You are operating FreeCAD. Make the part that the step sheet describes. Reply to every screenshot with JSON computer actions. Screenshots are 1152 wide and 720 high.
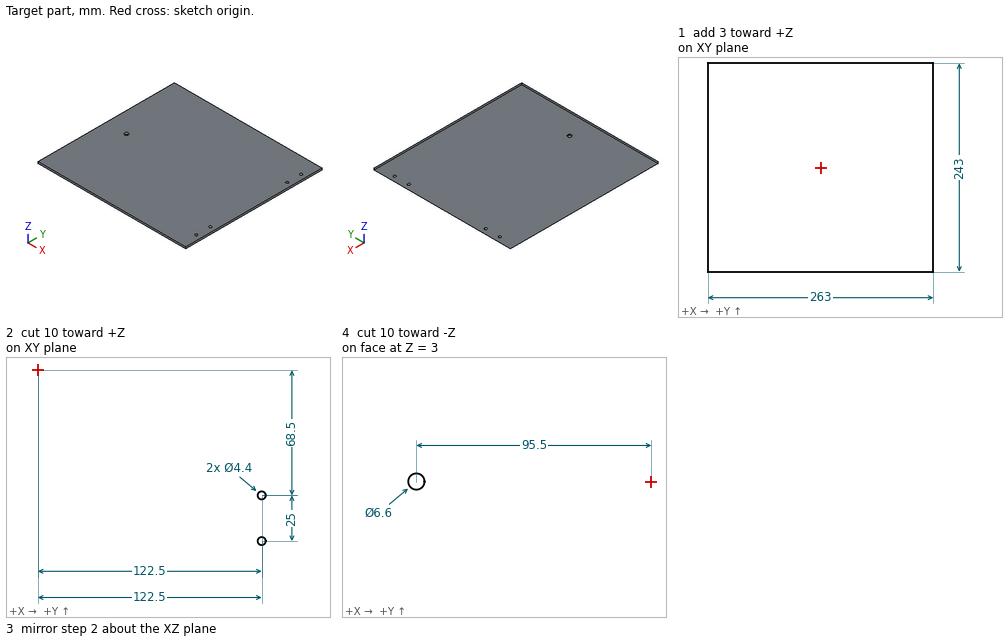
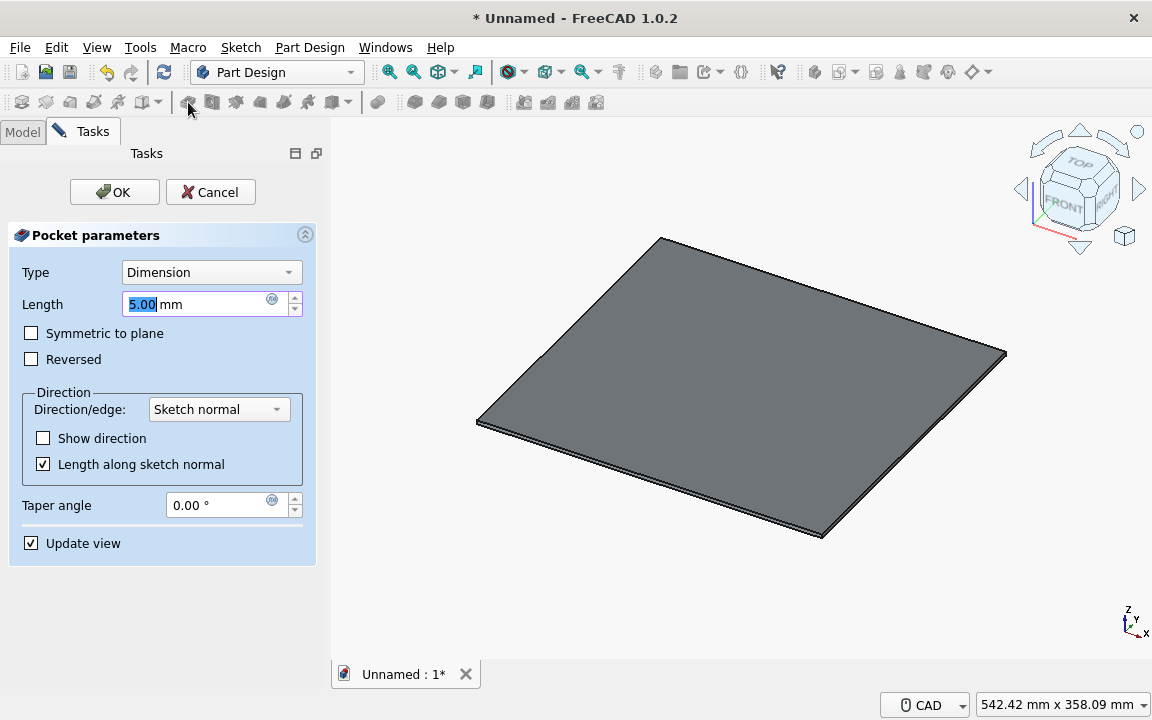
{"action": "type", "text": "10"}
{"action": "key", "text": "Tab"}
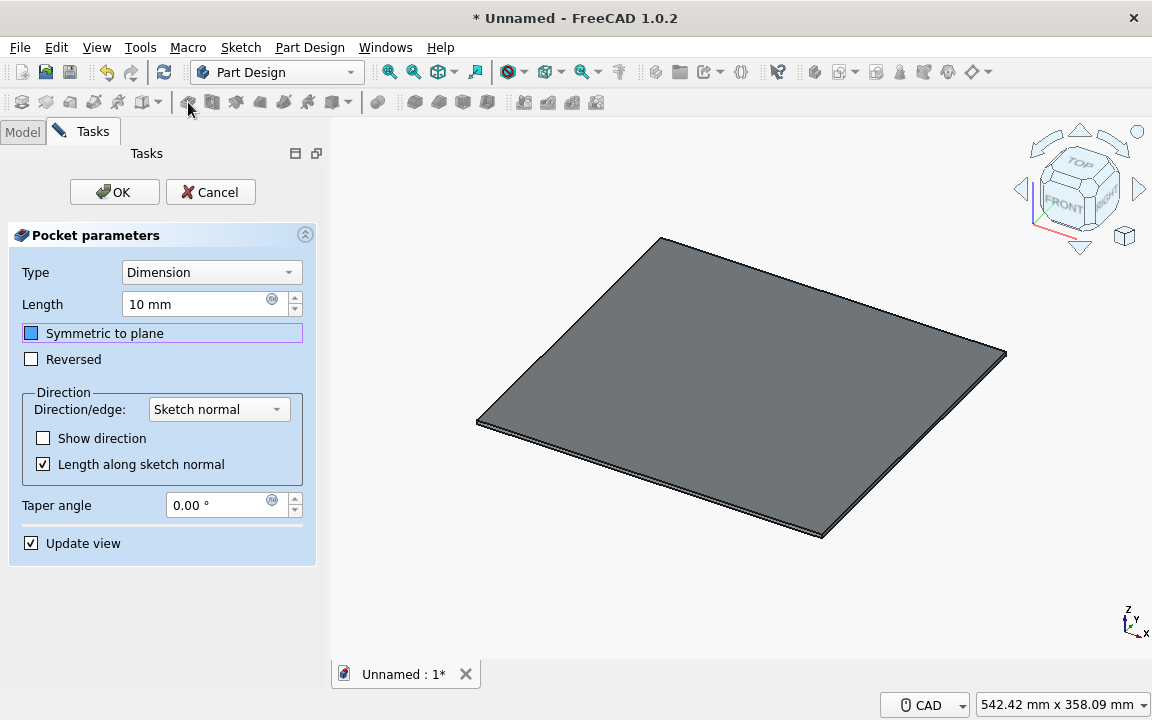
{"action": "left_click", "coordinate": [30, 359]}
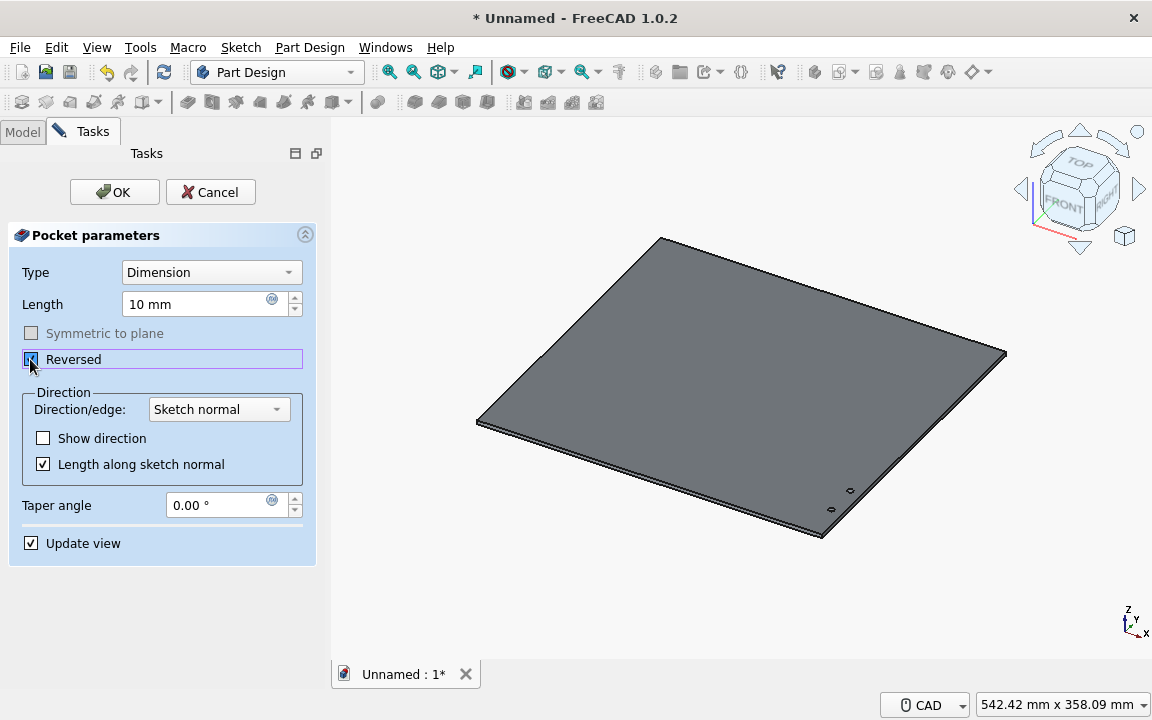
{"action": "left_click", "coordinate": [115, 192]}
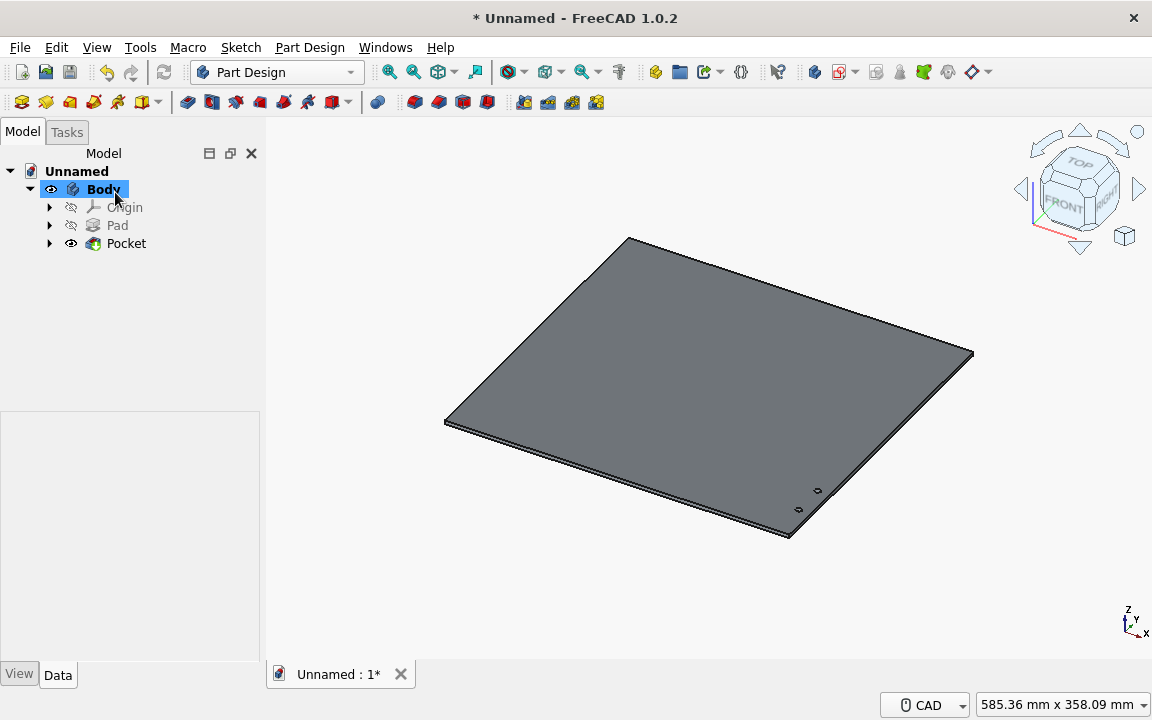
{"action": "left_click", "coordinate": [116, 243]}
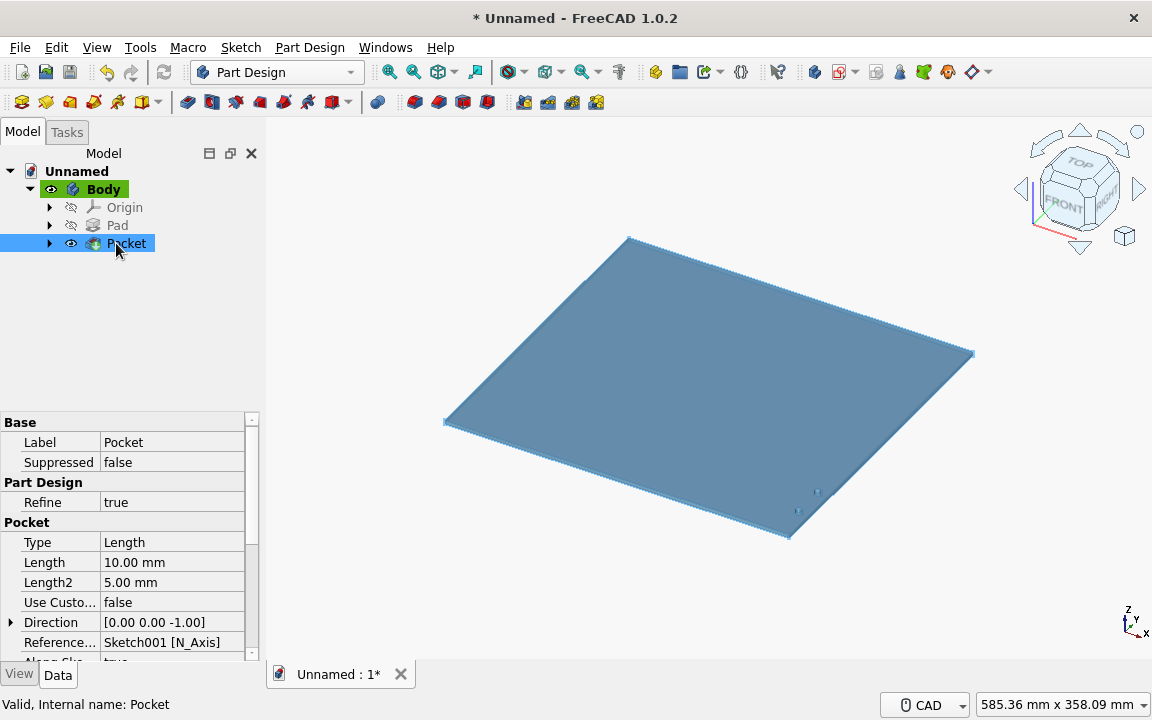
{"action": "left_click", "coordinate": [524, 102]}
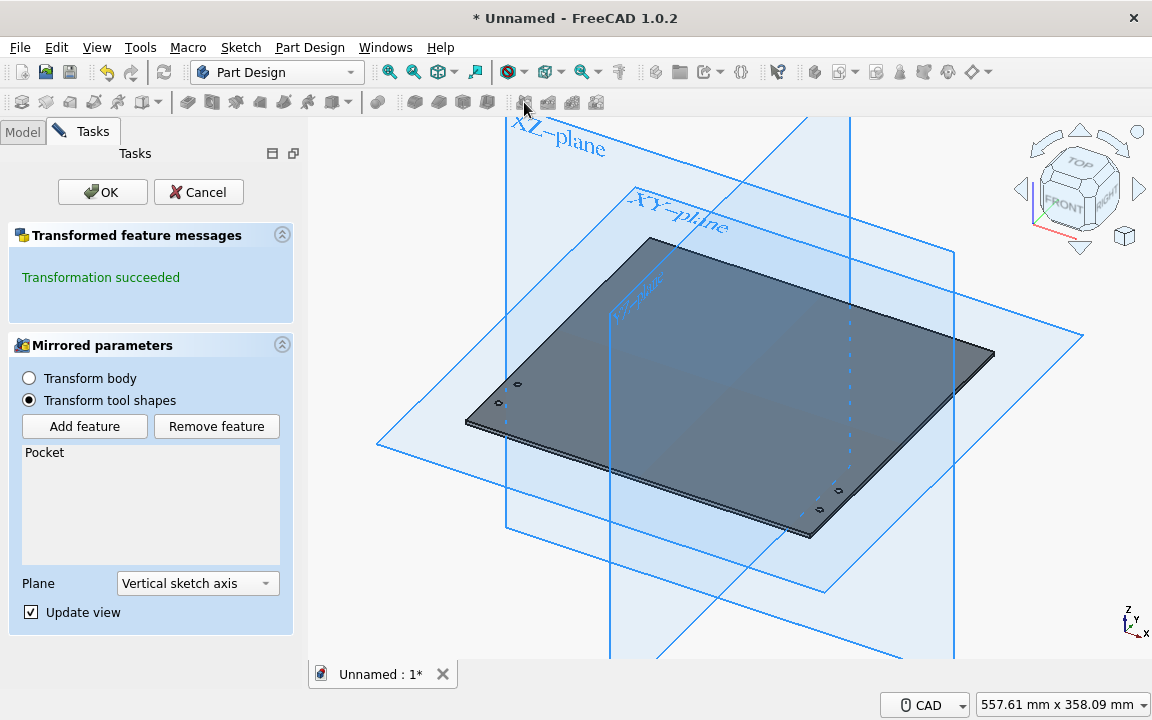
{"action": "left_click", "coordinate": [198, 584]}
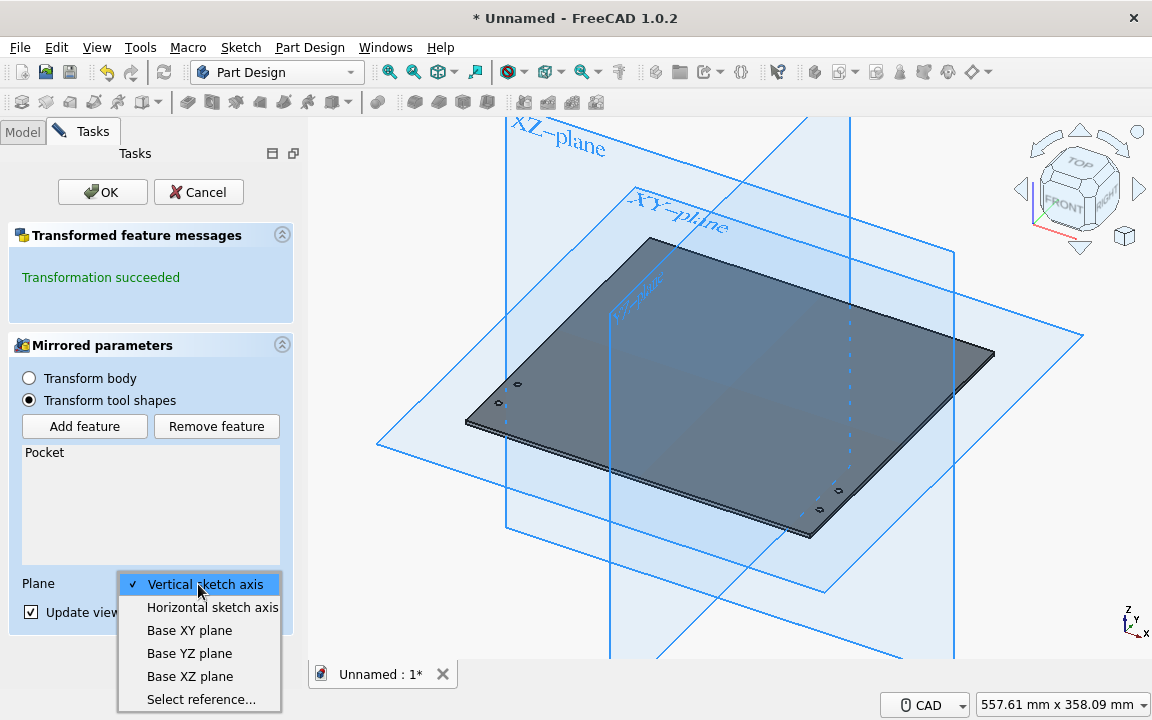
{"action": "left_click", "coordinate": [198, 676]}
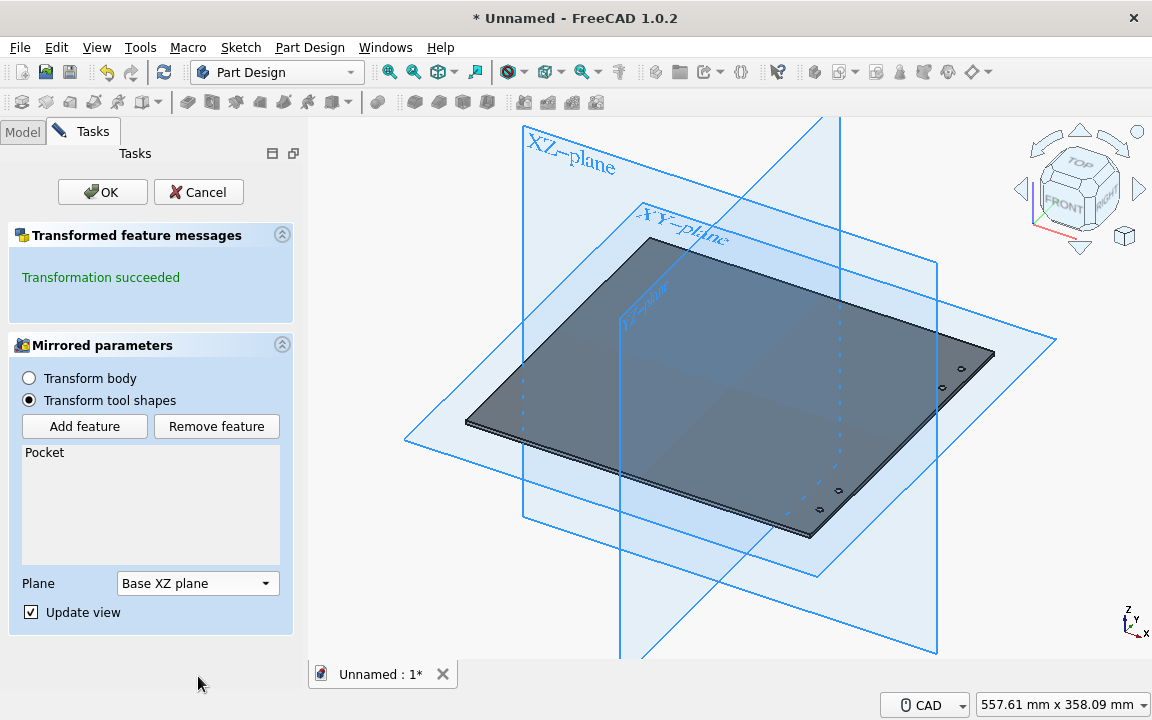
{"action": "left_click", "coordinate": [103, 192]}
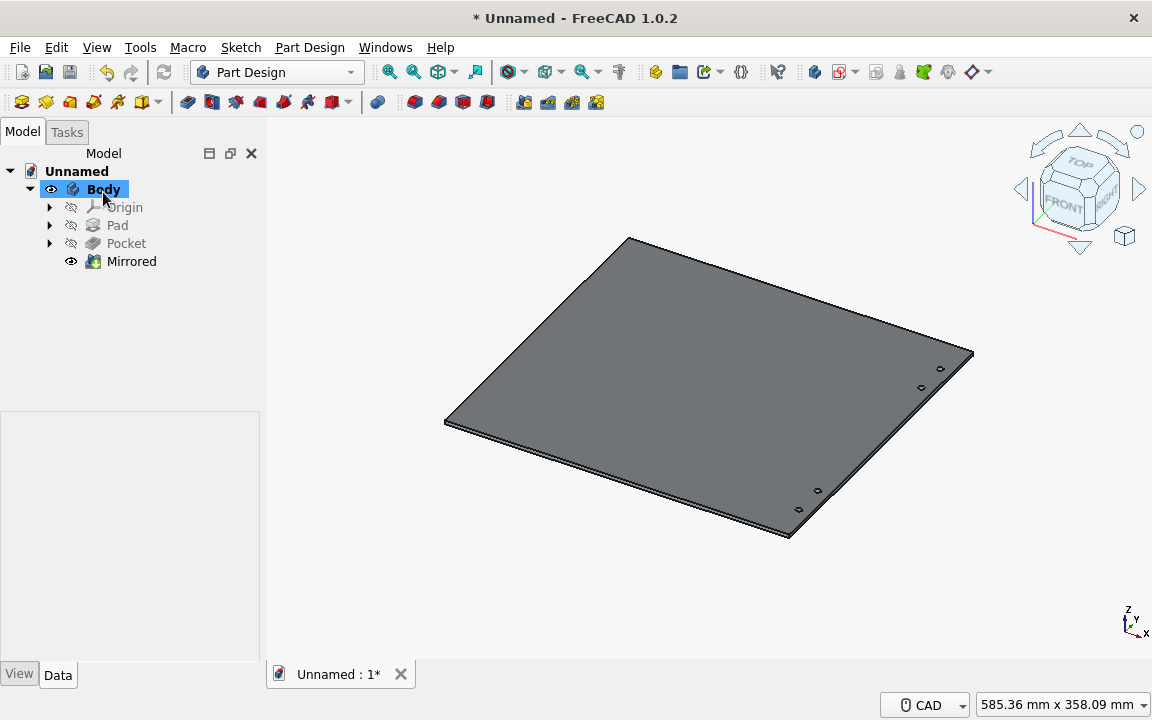
{"action": "left_click", "coordinate": [709, 385]}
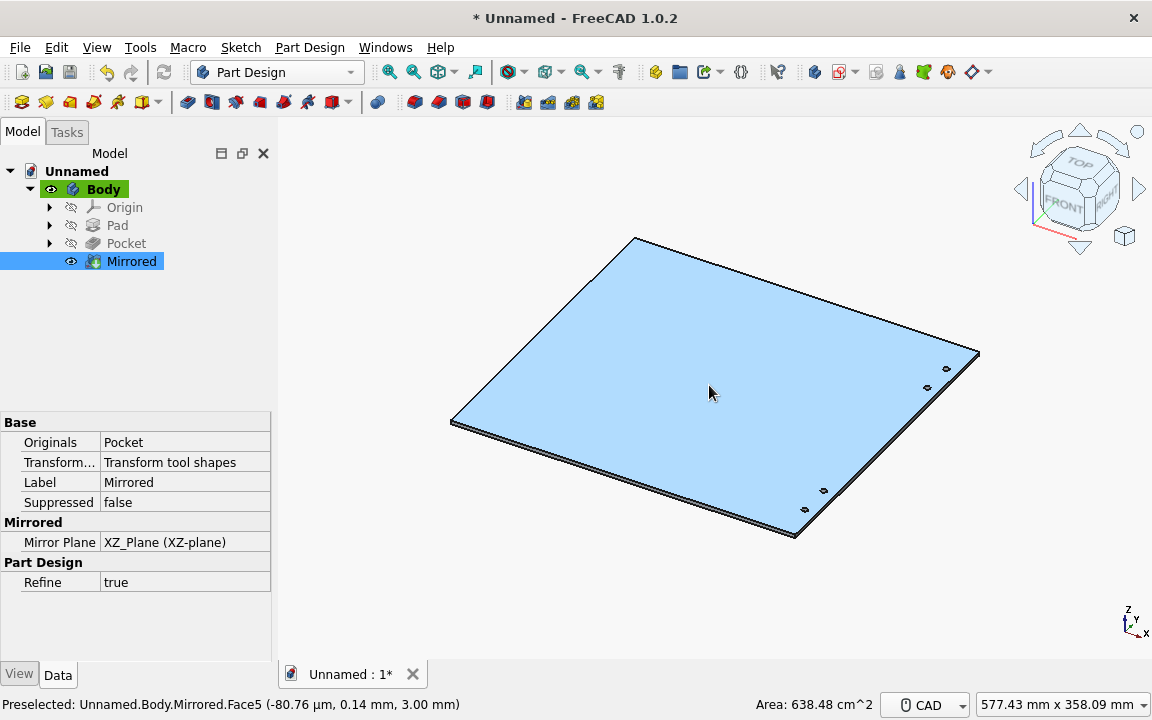
{"action": "left_click", "coordinate": [840, 72]}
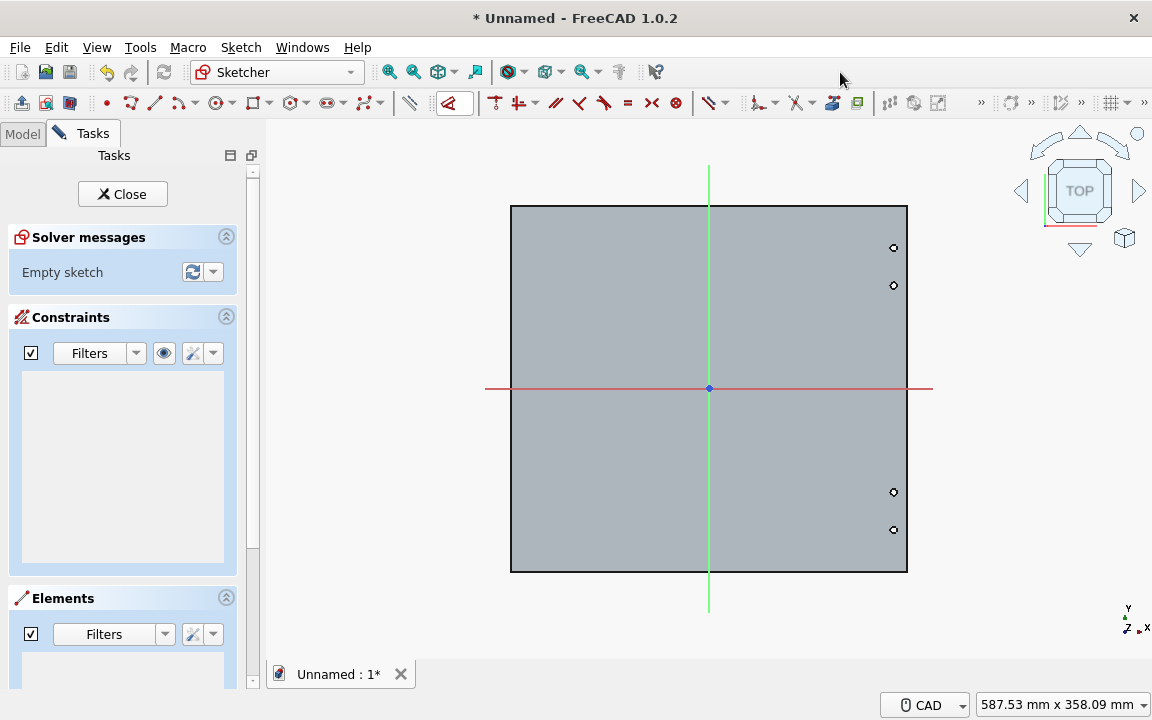
{"action": "scroll", "coordinate": [561, 389], "scroll_direction": "up", "scroll_amount": 15}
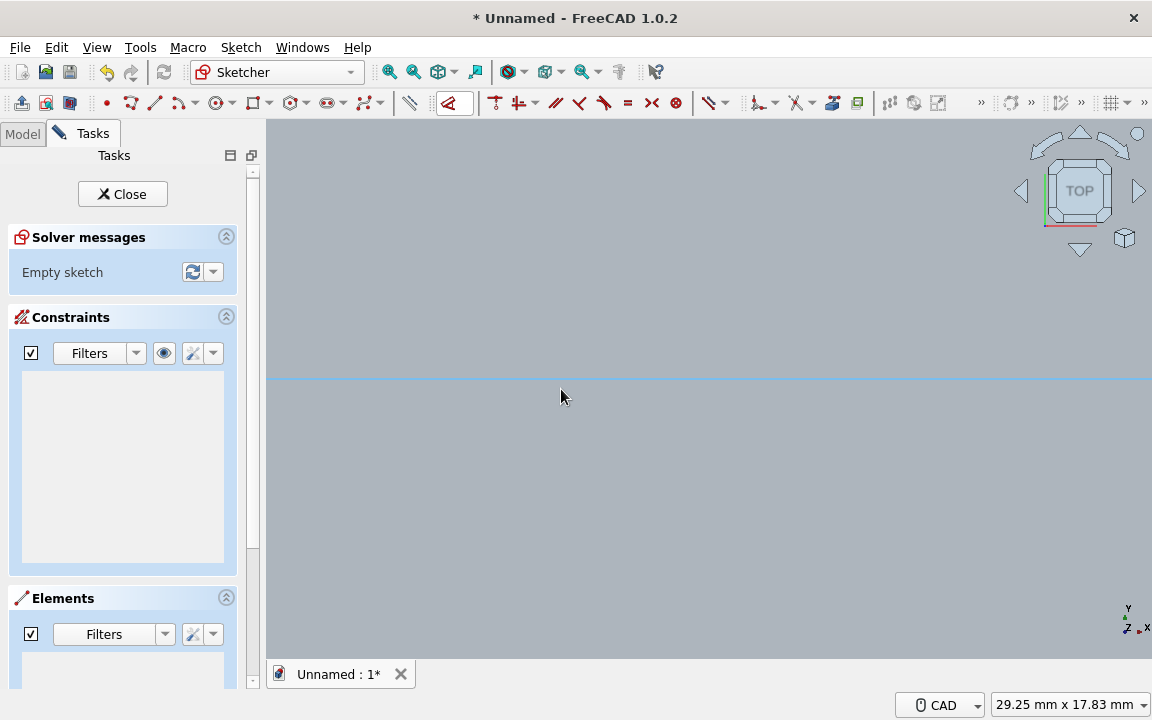
{"action": "scroll", "coordinate": [628, 368], "scroll_direction": "up", "scroll_amount": 3}